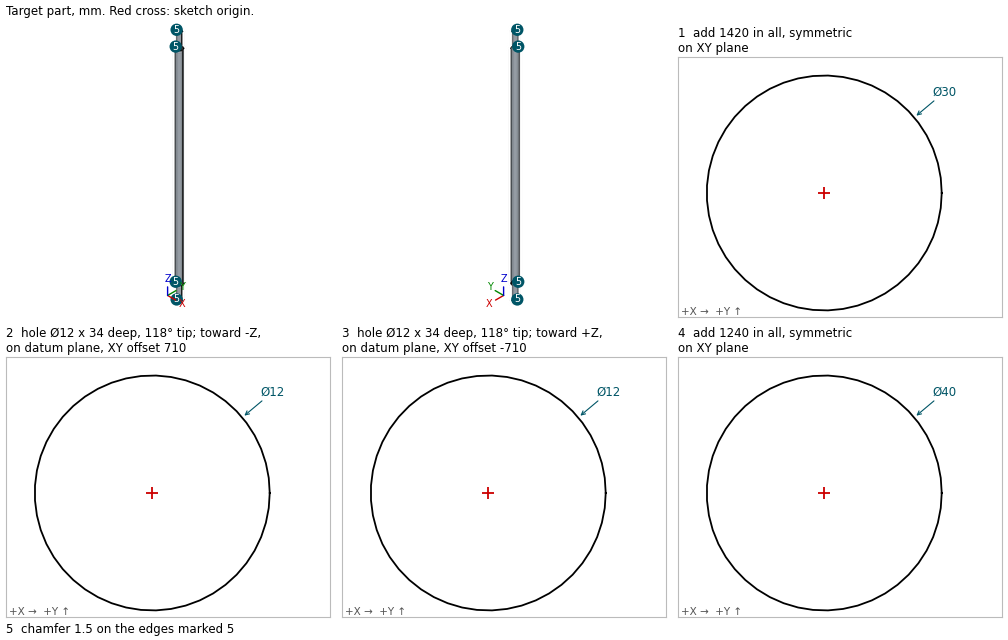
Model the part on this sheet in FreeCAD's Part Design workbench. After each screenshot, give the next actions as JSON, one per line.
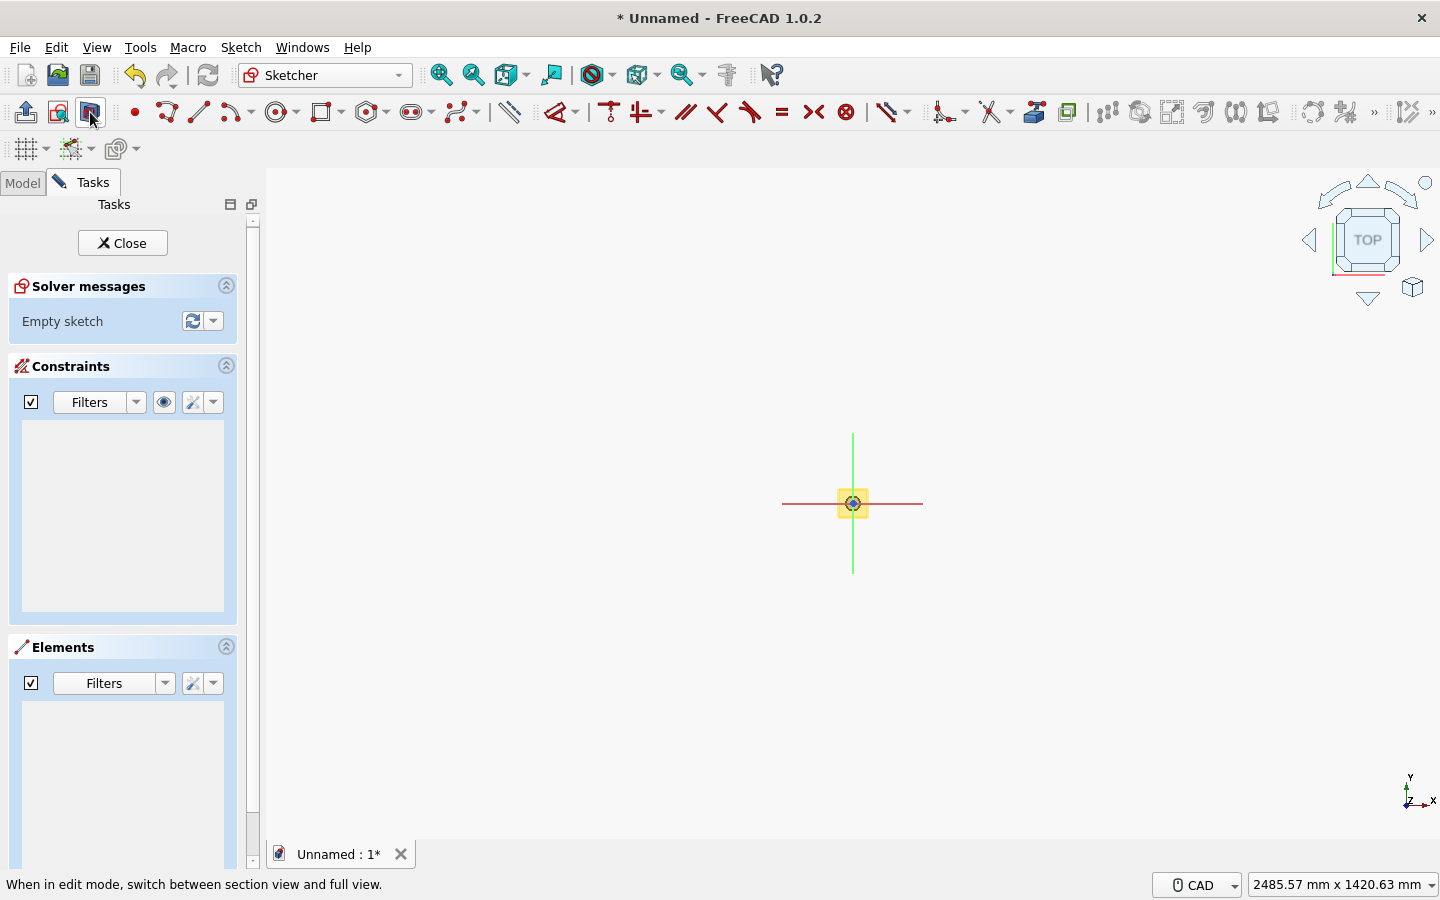
{"action": "scroll", "coordinate": [857, 504], "scroll_direction": "up", "scroll_amount": 15}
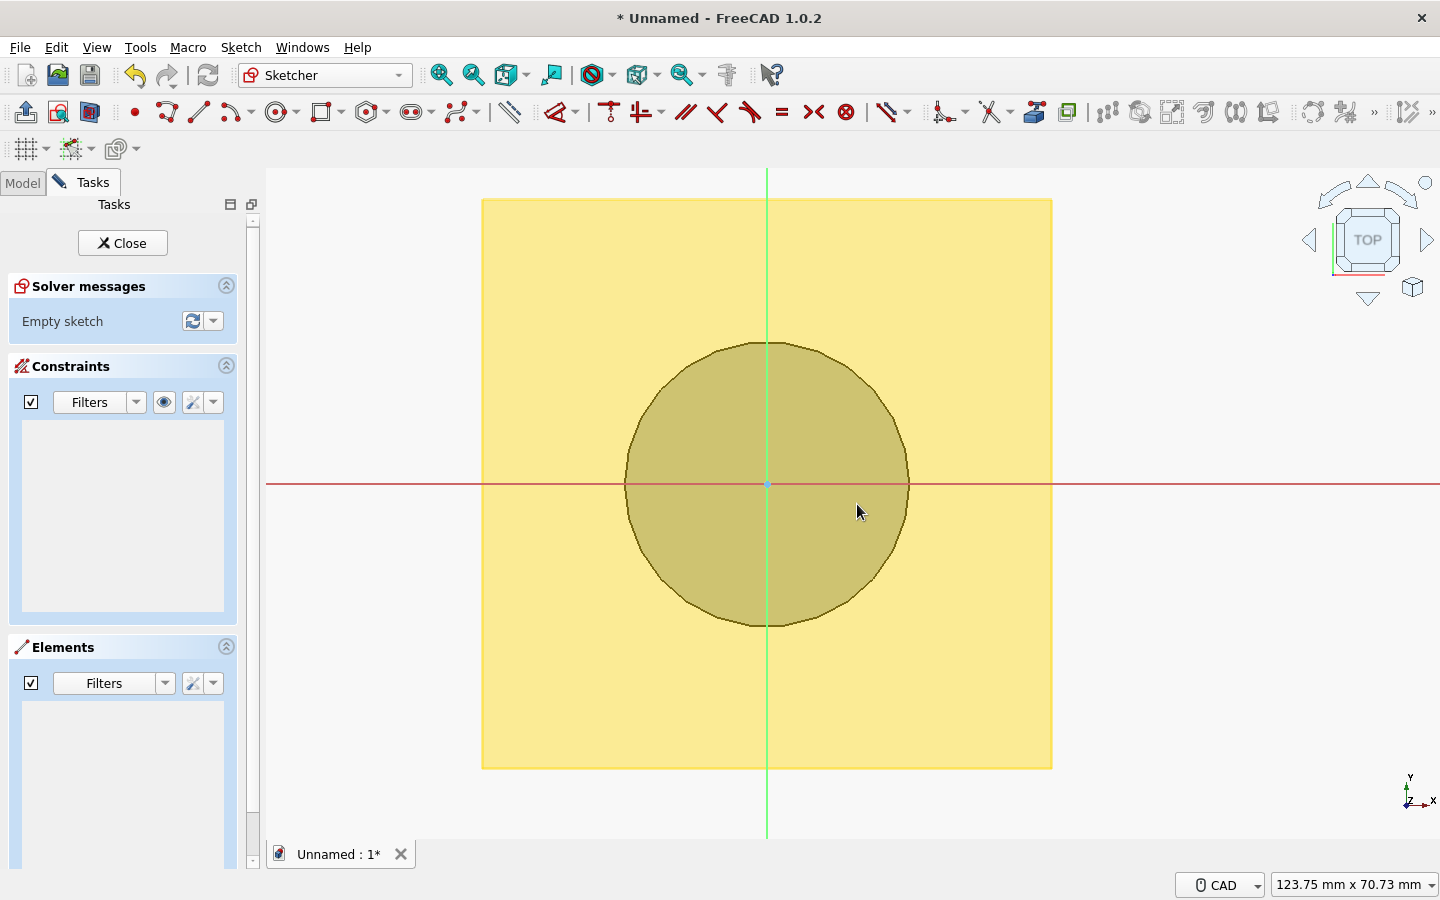
{"action": "scroll", "coordinate": [761, 478], "scroll_direction": "up", "scroll_amount": 7}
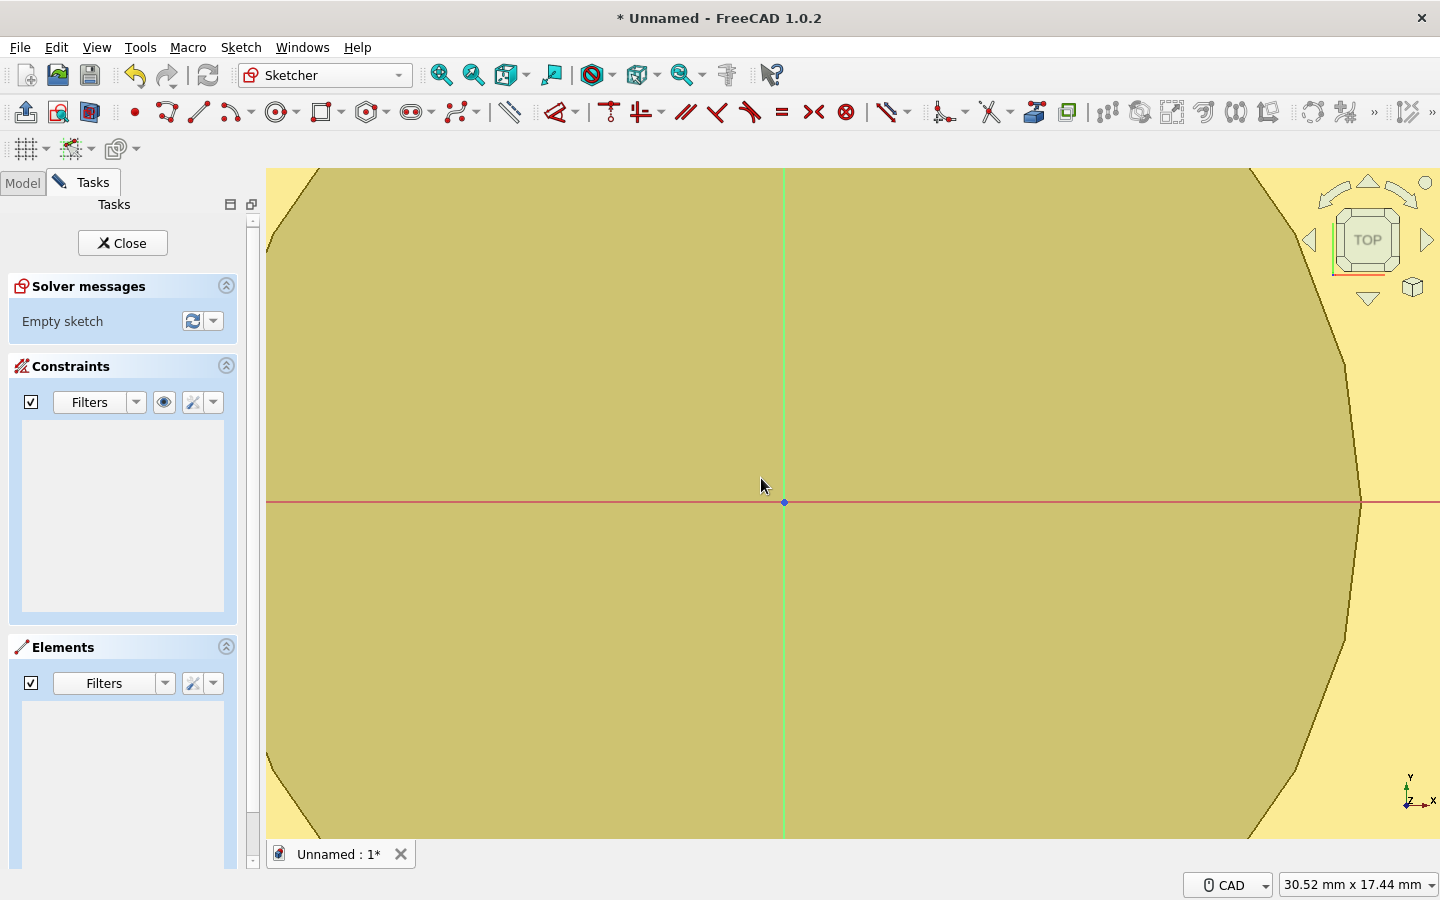
{"action": "left_click", "coordinate": [276, 112]}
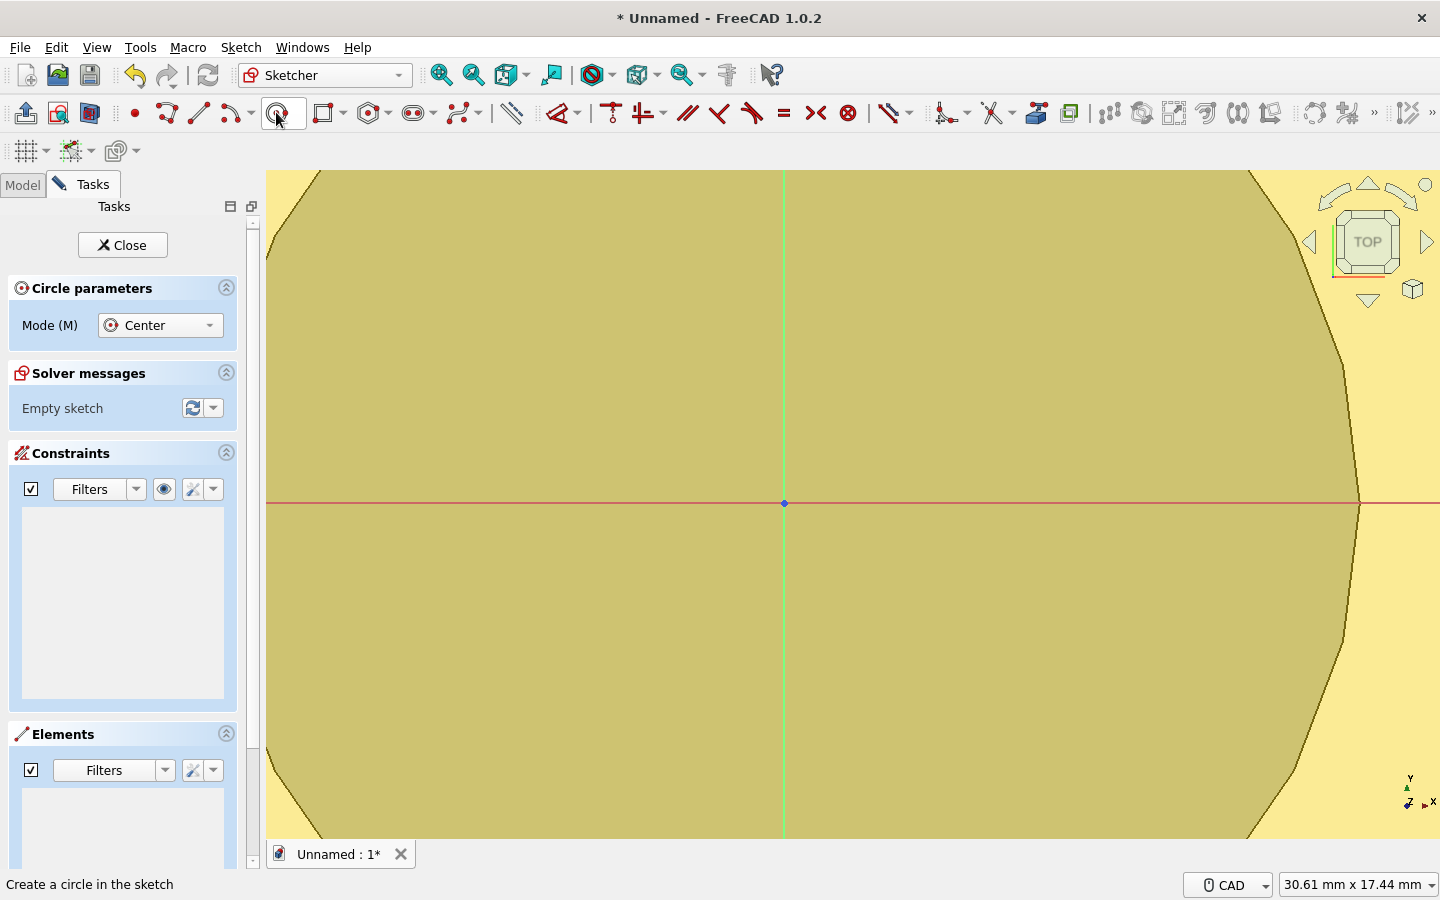
{"action": "left_click", "coordinate": [784, 503]}
{"action": "mouse_move", "coordinate": [947, 341]}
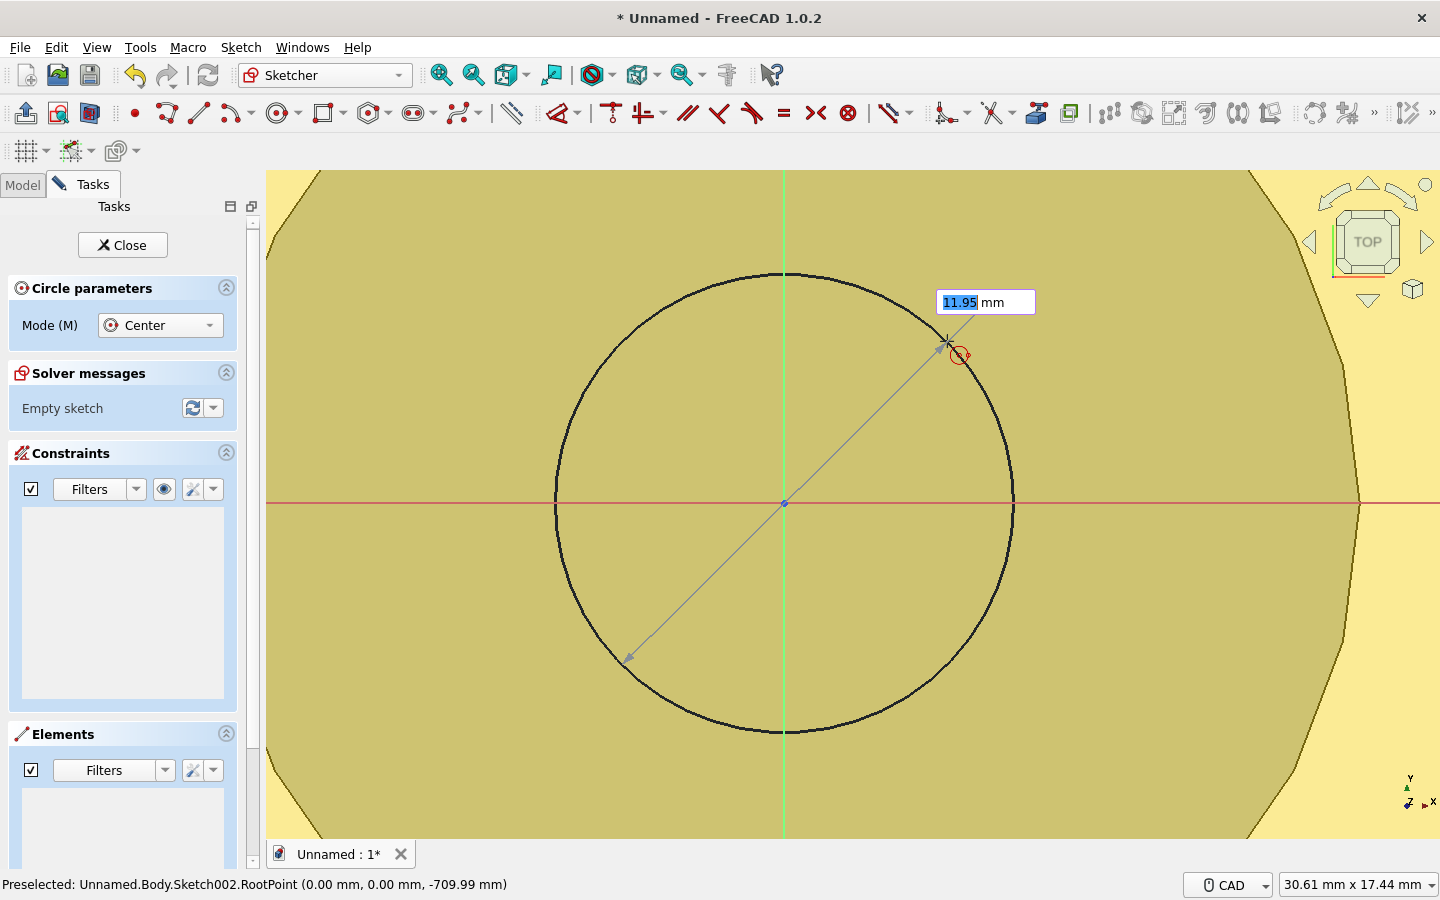
{"action": "type", "text": "12"}
{"action": "key", "text": "Return"}
{"action": "key", "text": "Escape"}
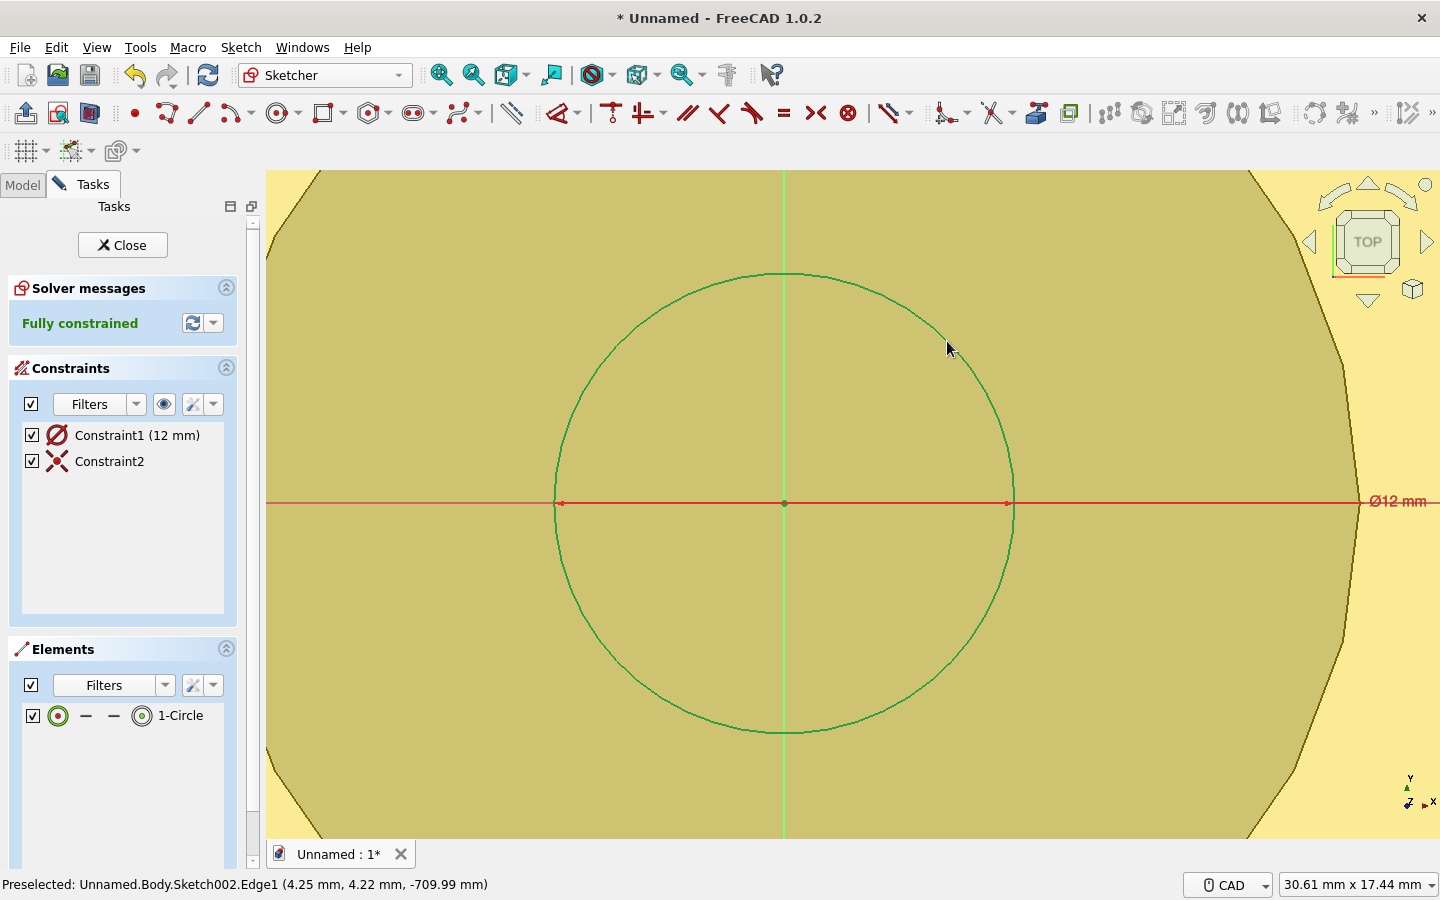
{"action": "left_click", "coordinate": [123, 245]}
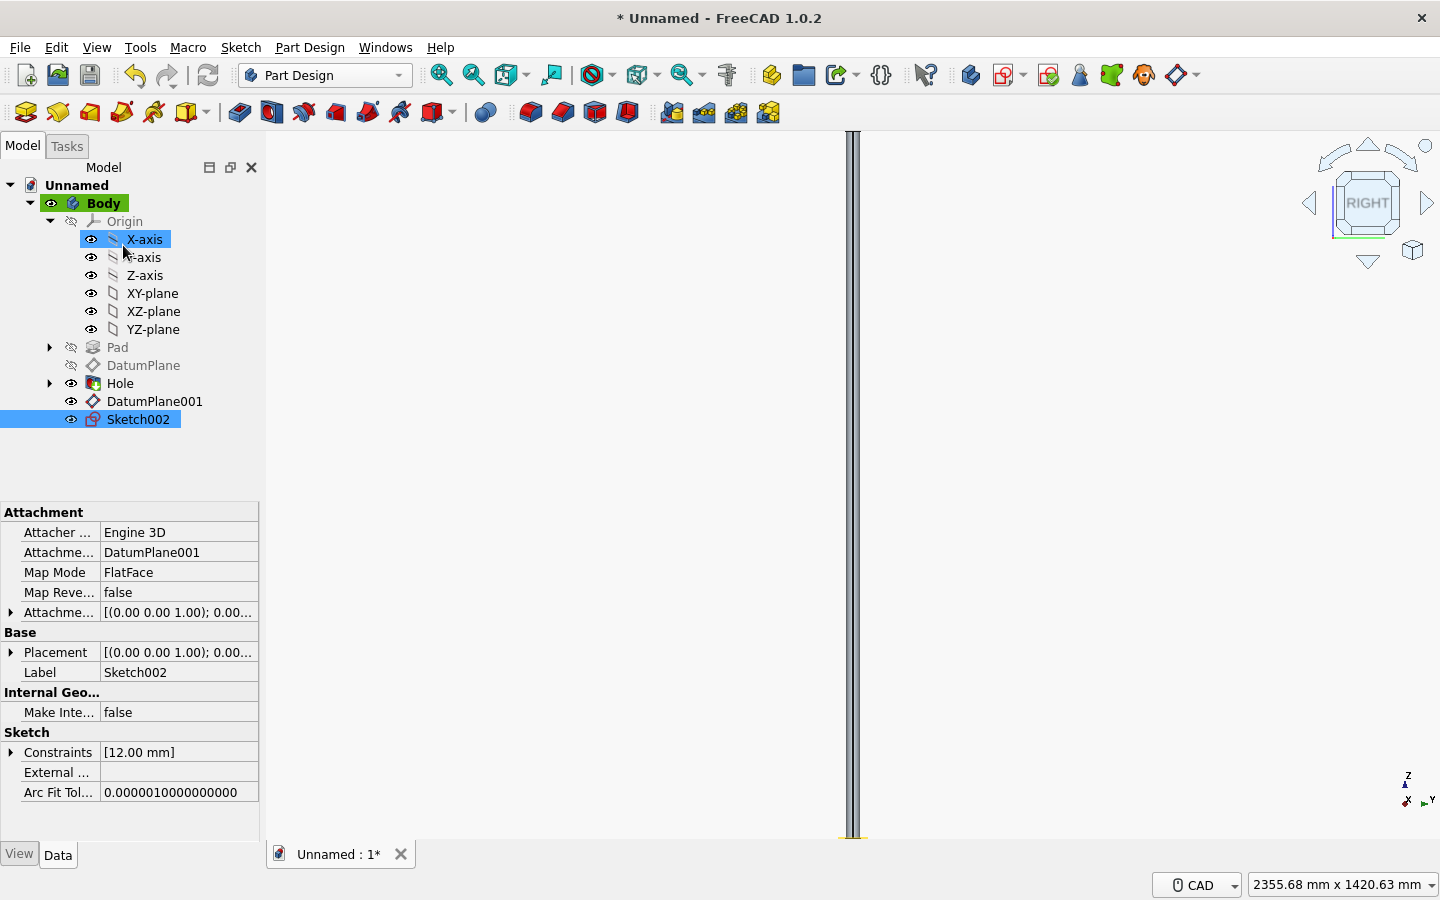
{"action": "left_click", "coordinate": [272, 112]}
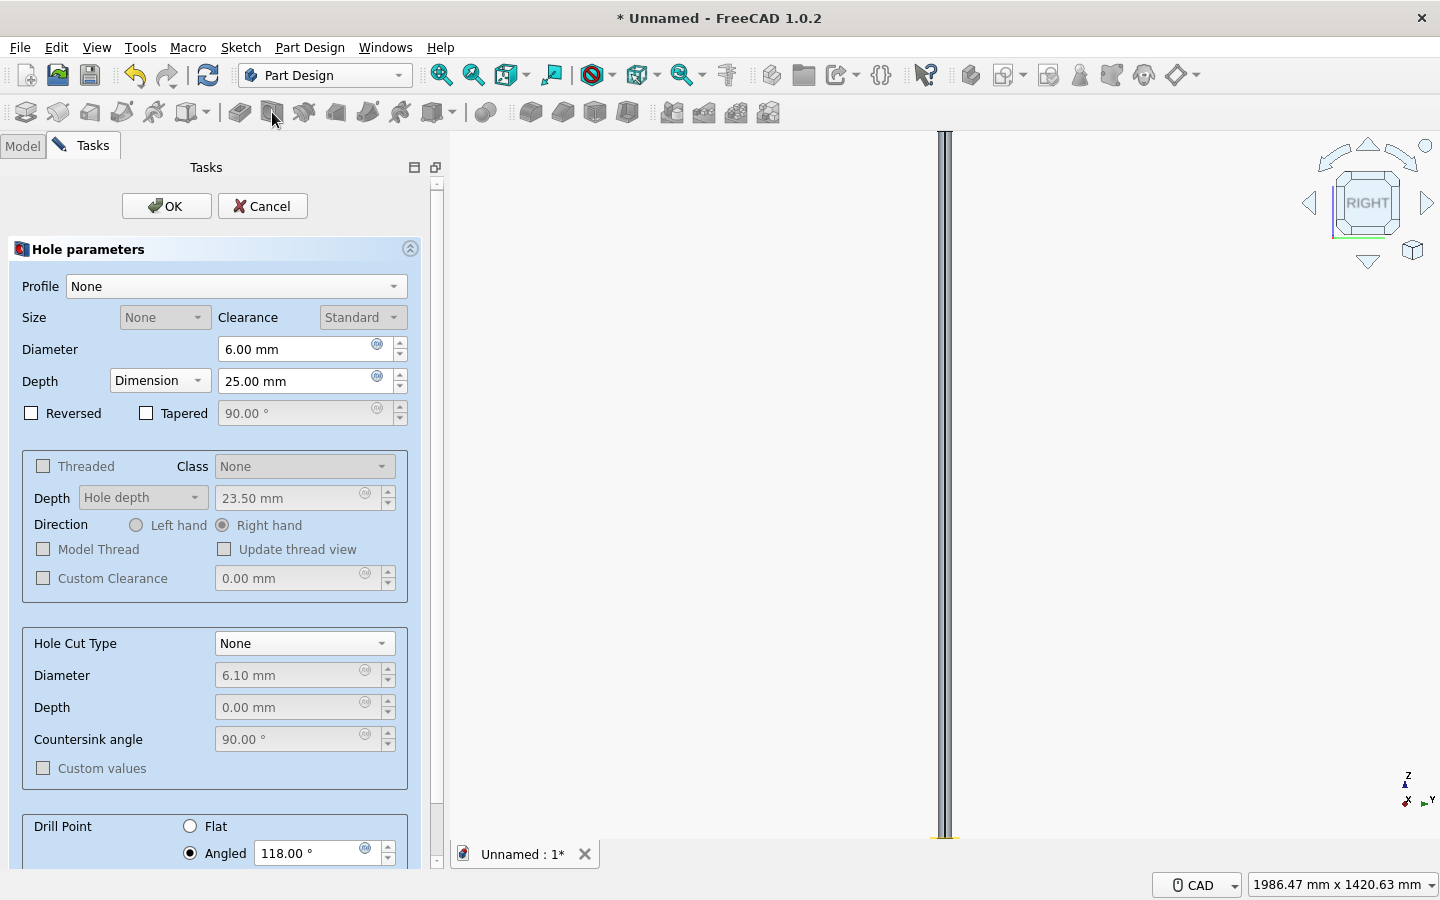
{"action": "triple_click", "coordinate": [305, 349]}